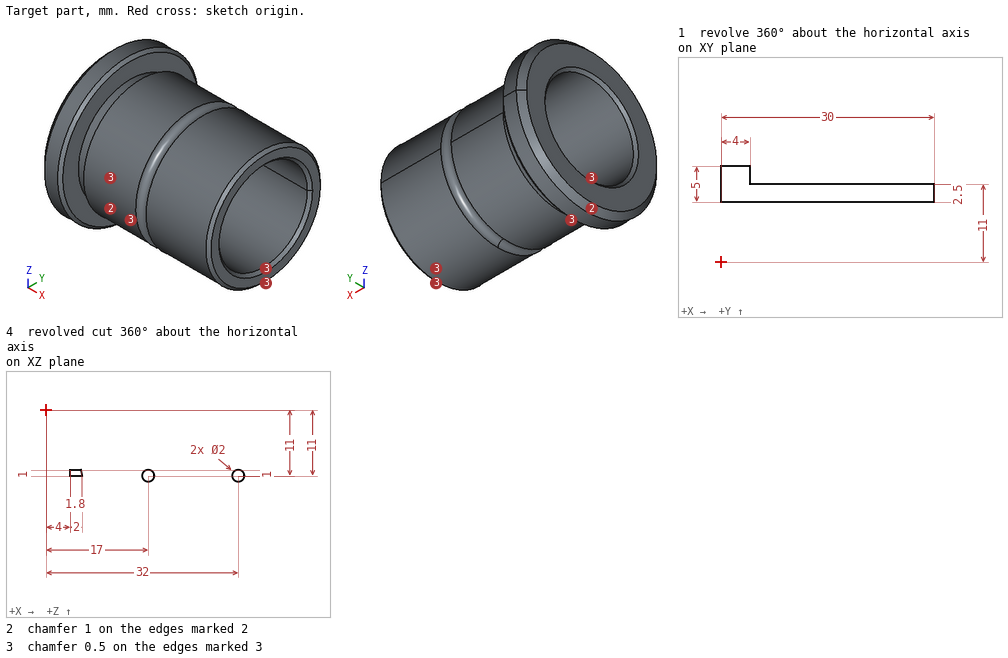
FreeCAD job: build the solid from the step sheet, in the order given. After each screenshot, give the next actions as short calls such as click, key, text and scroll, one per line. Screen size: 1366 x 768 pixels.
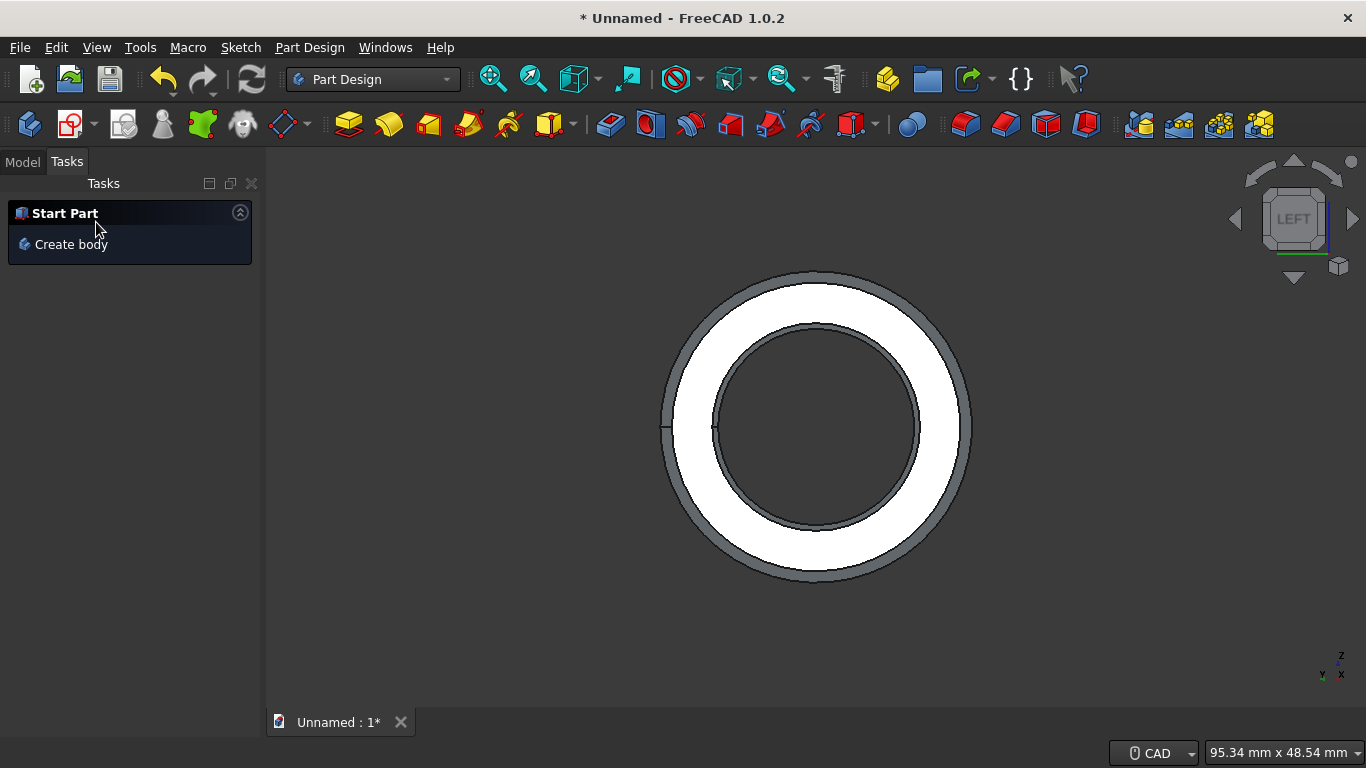
click(70, 124)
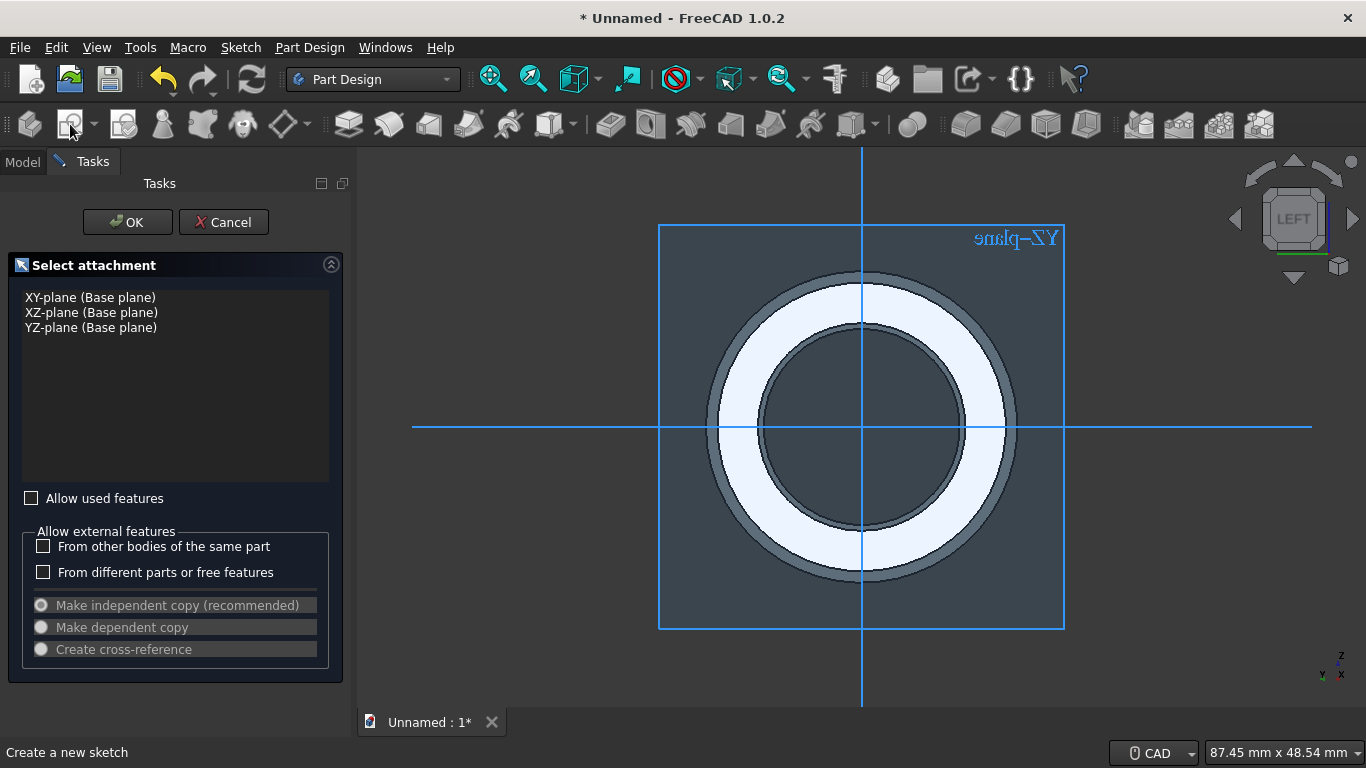
click(82, 312)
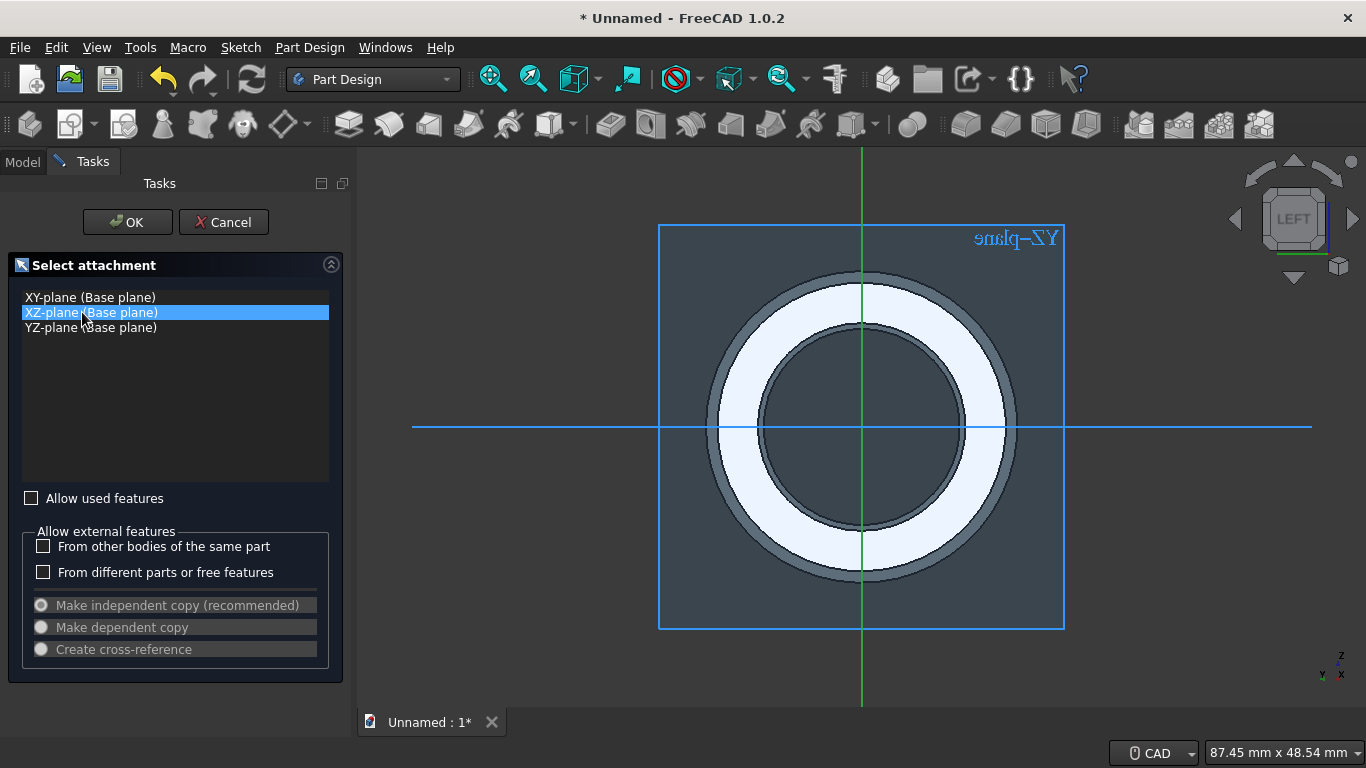
click(128, 222)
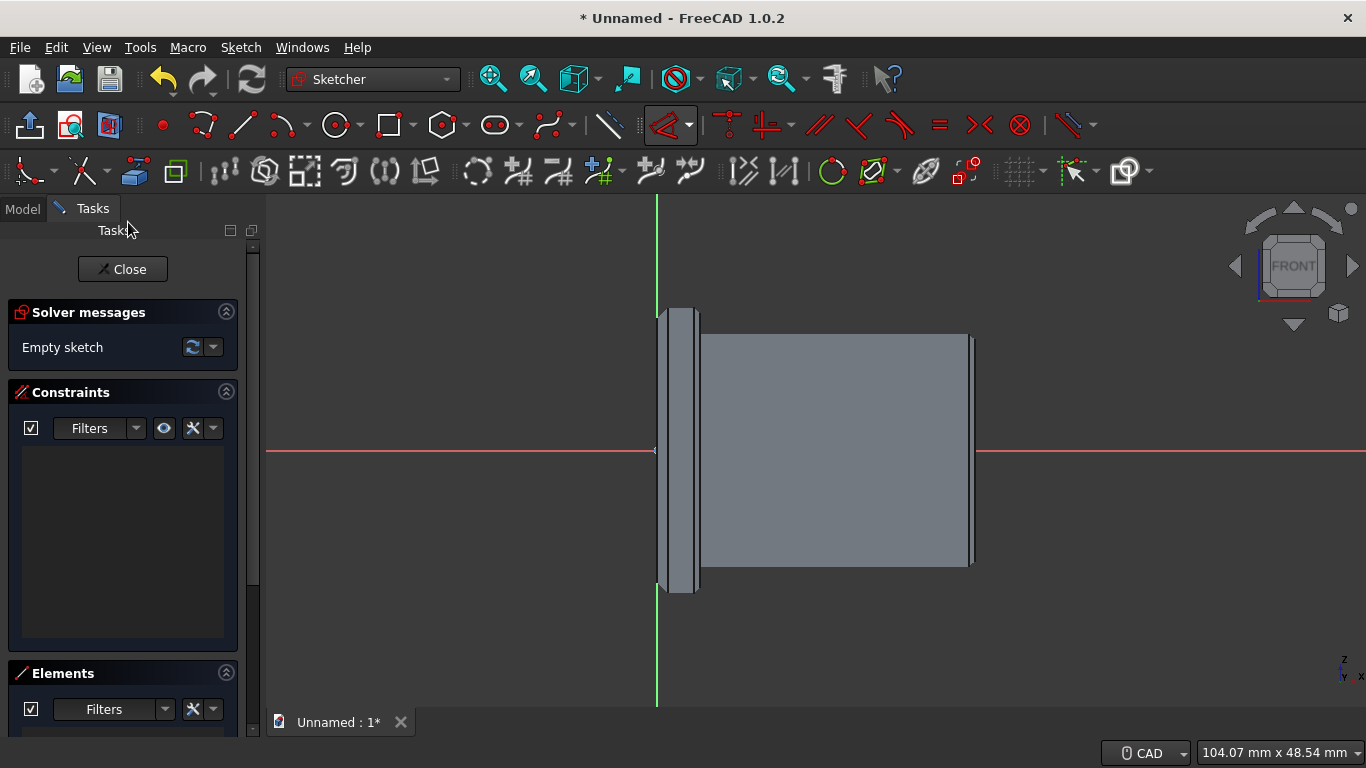
click(110, 126)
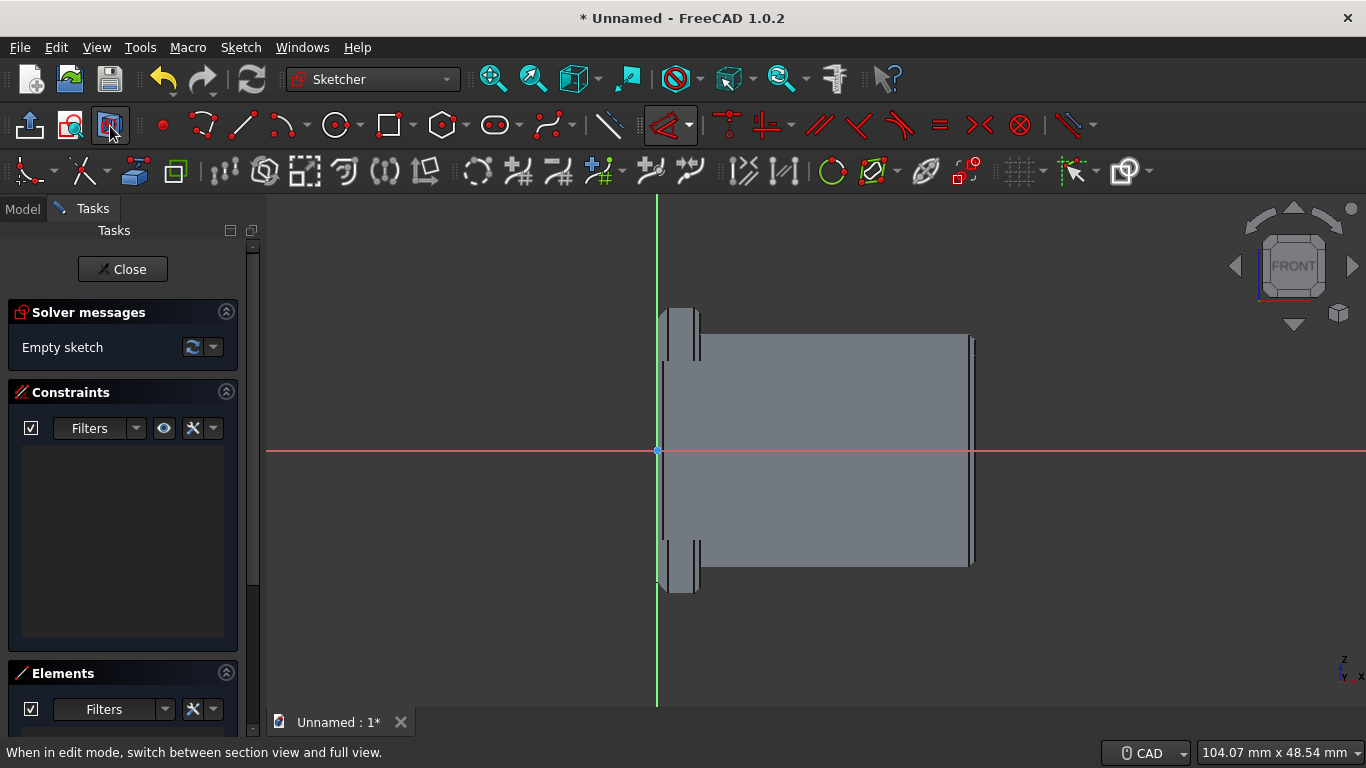
scroll(934, 591, up, 3)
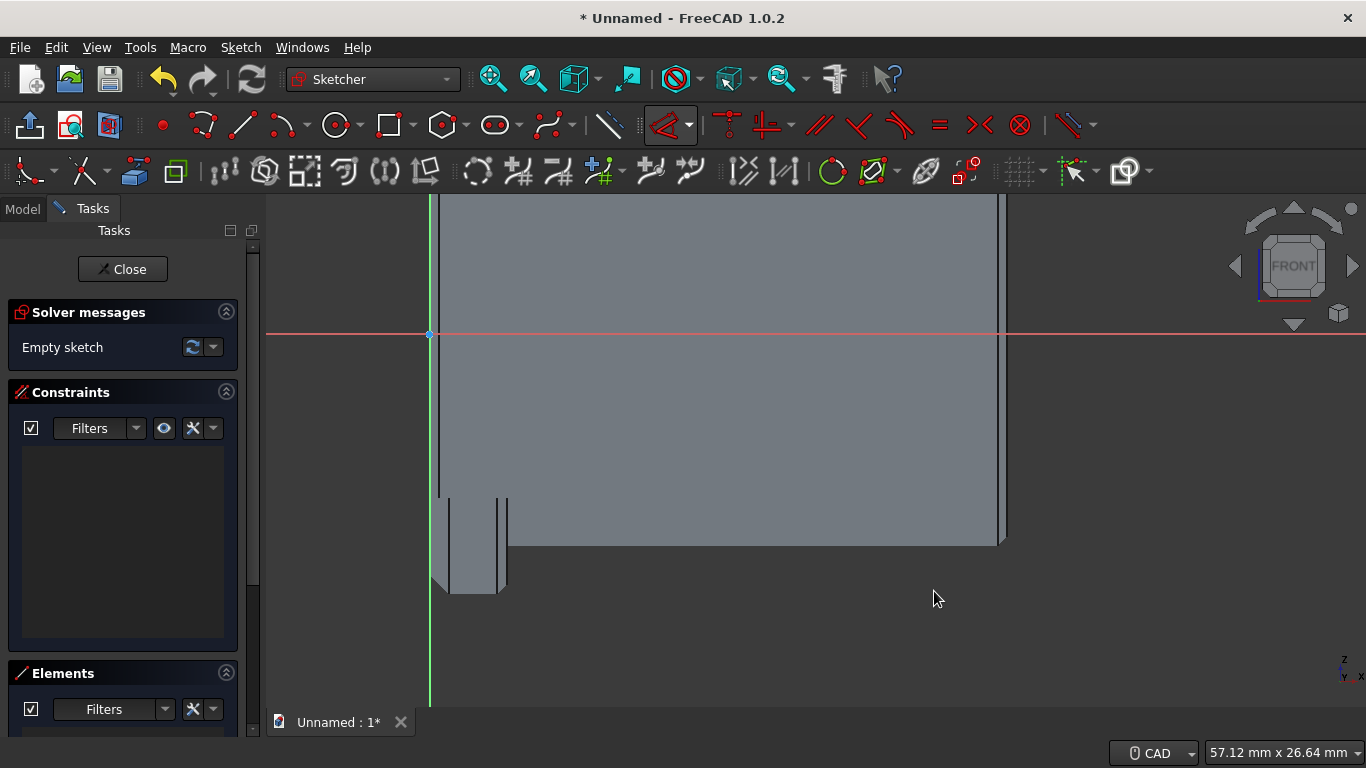
click(204, 126)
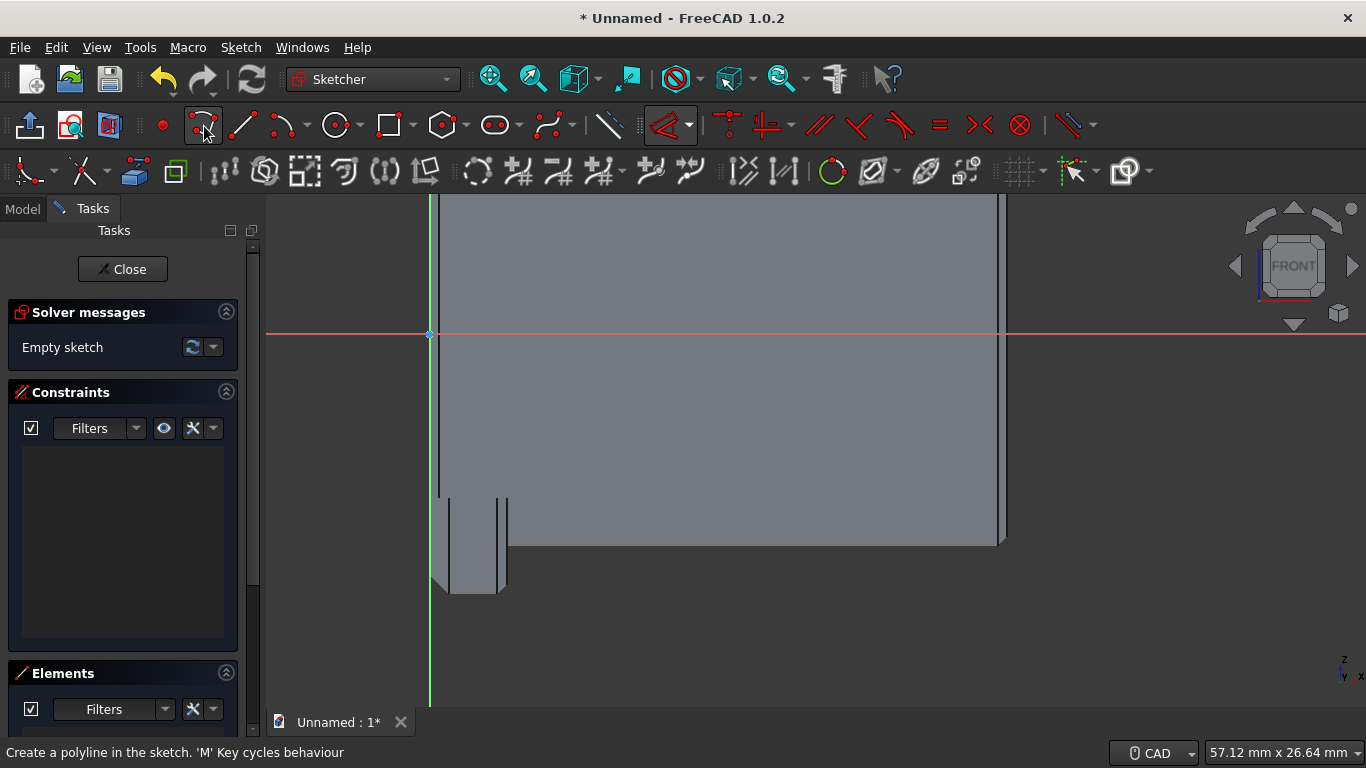
click(507, 527)
click(541, 527)
click(545, 546)
click(507, 546)
click(507, 528)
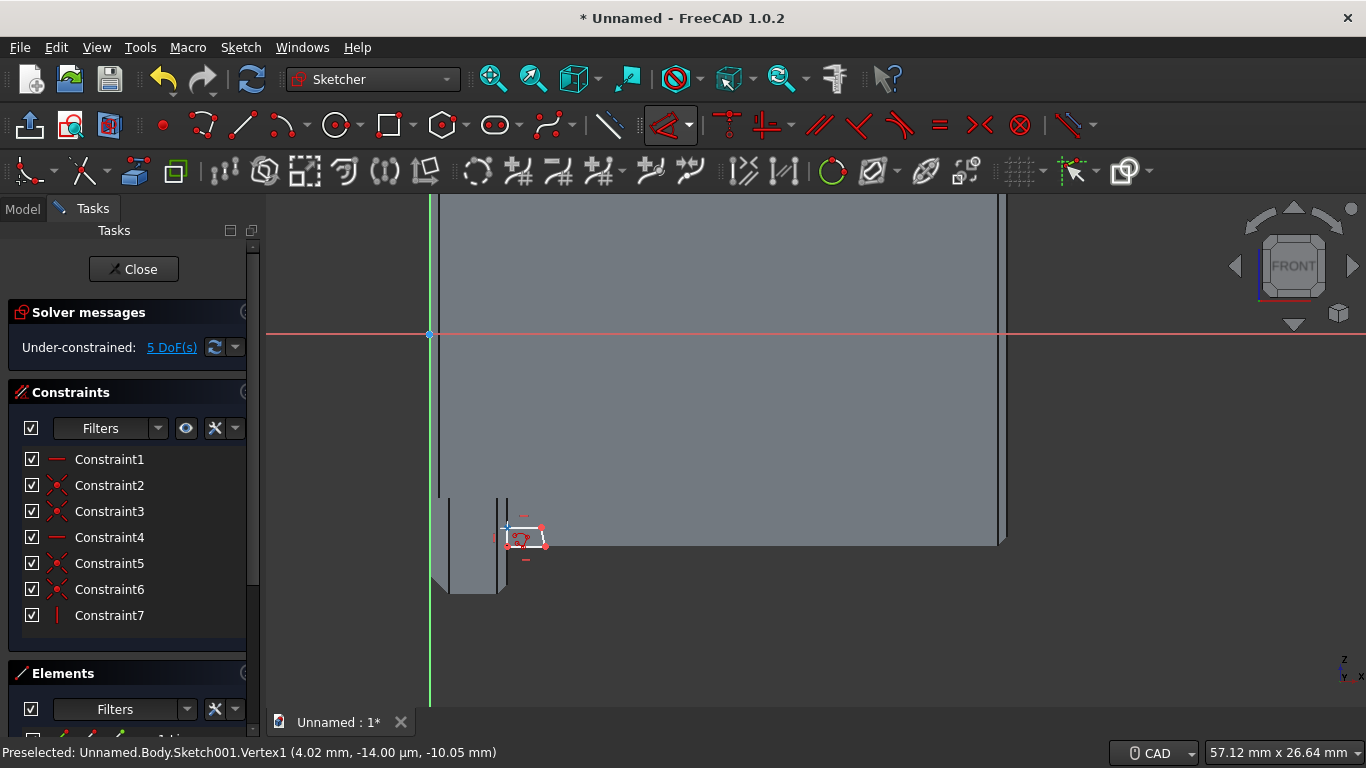
click(336, 126)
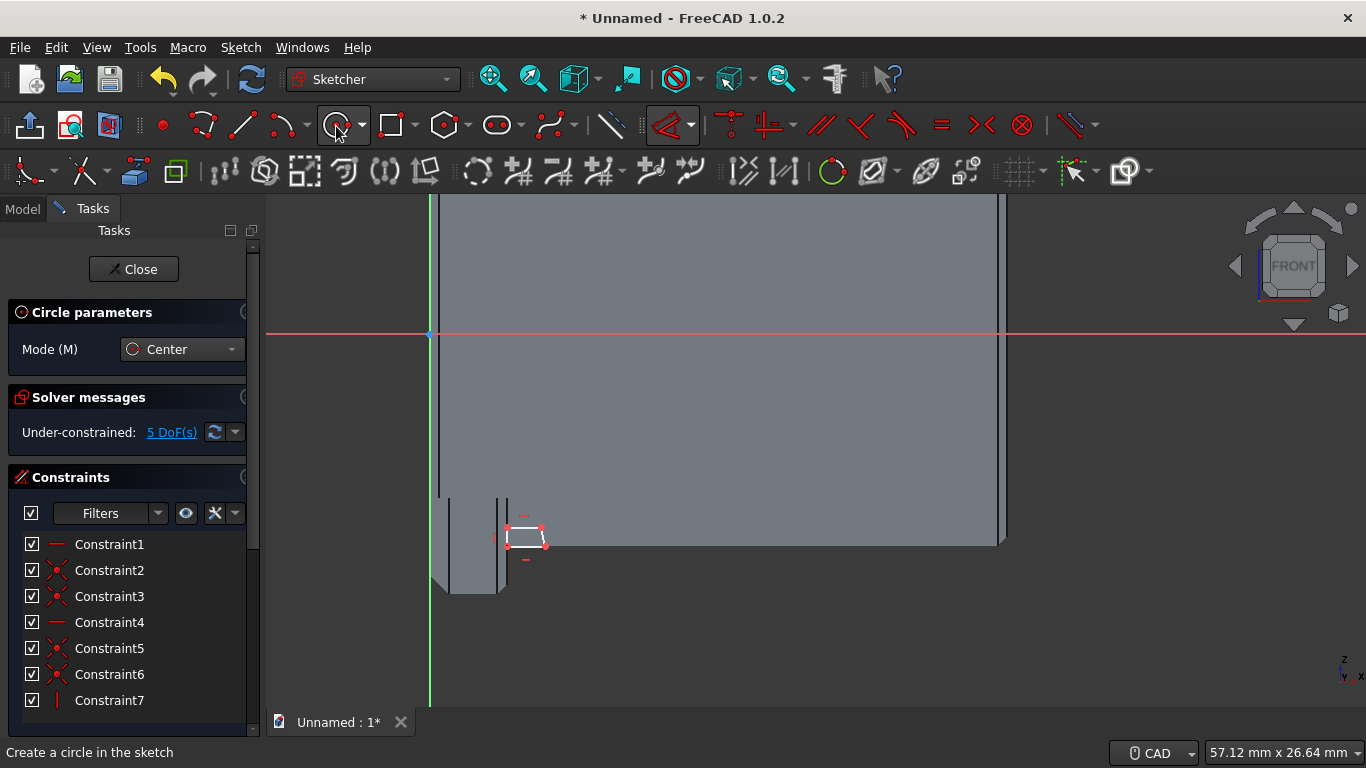
click(1046, 546)
move(1060, 533)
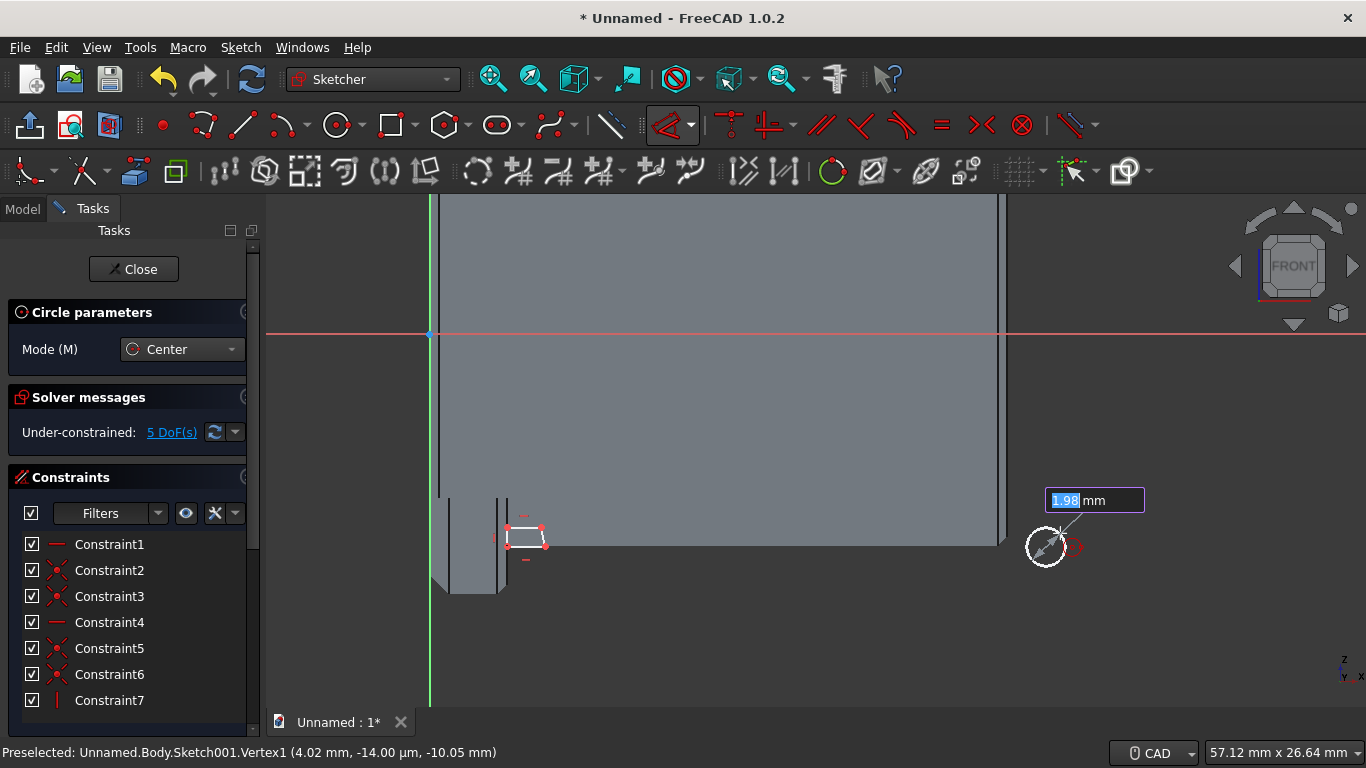
text(2)
key(Return)